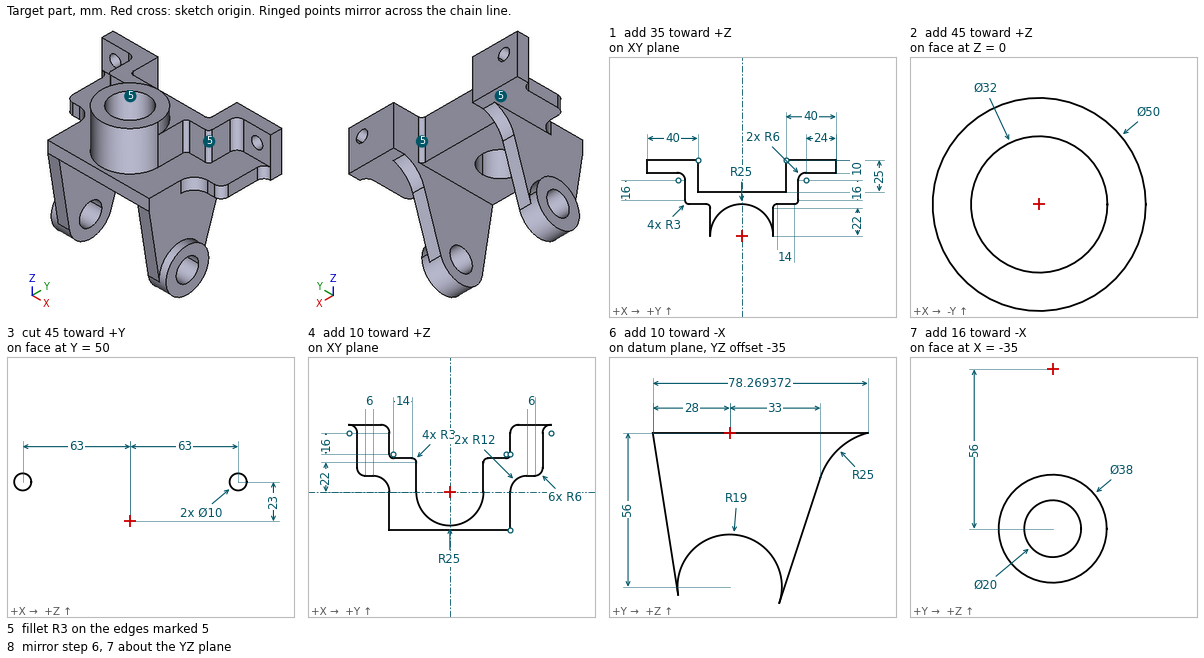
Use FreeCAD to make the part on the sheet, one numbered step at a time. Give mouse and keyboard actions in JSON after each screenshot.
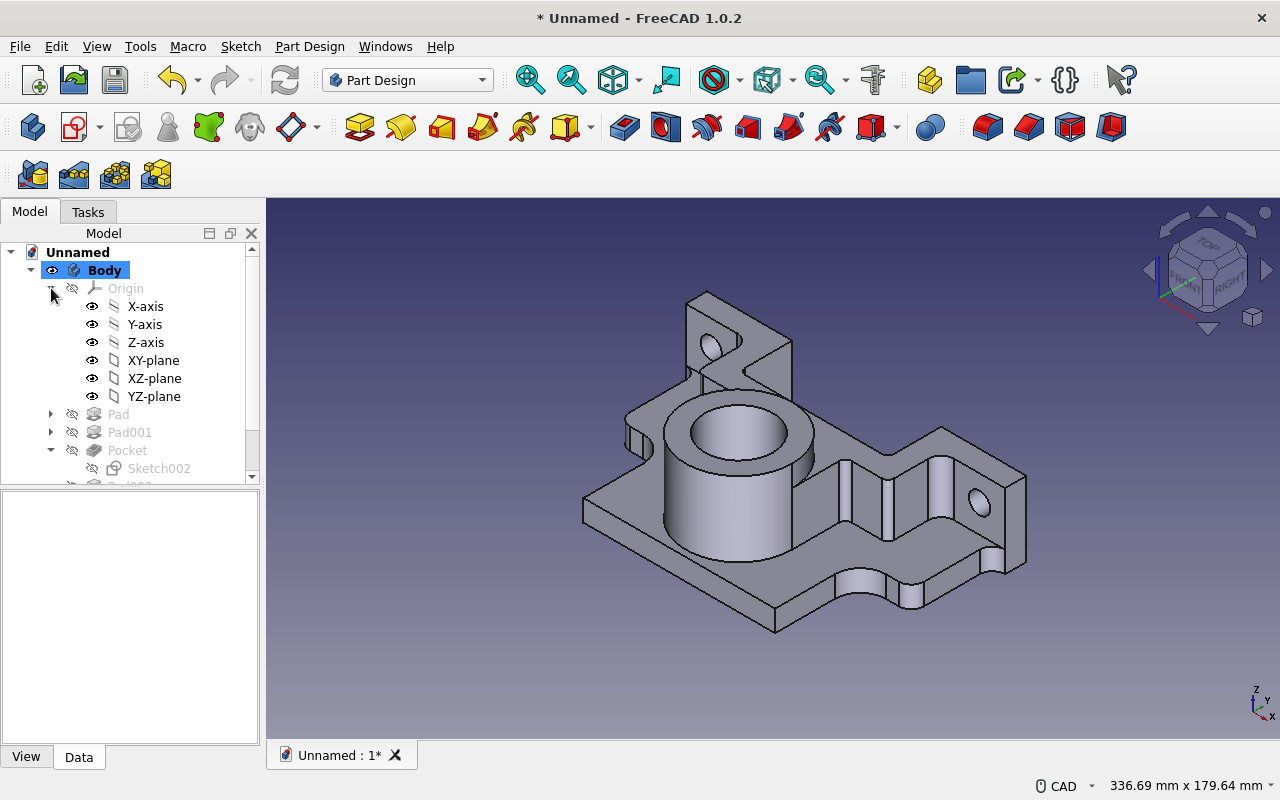
{"action": "left_click", "coordinate": [137, 396]}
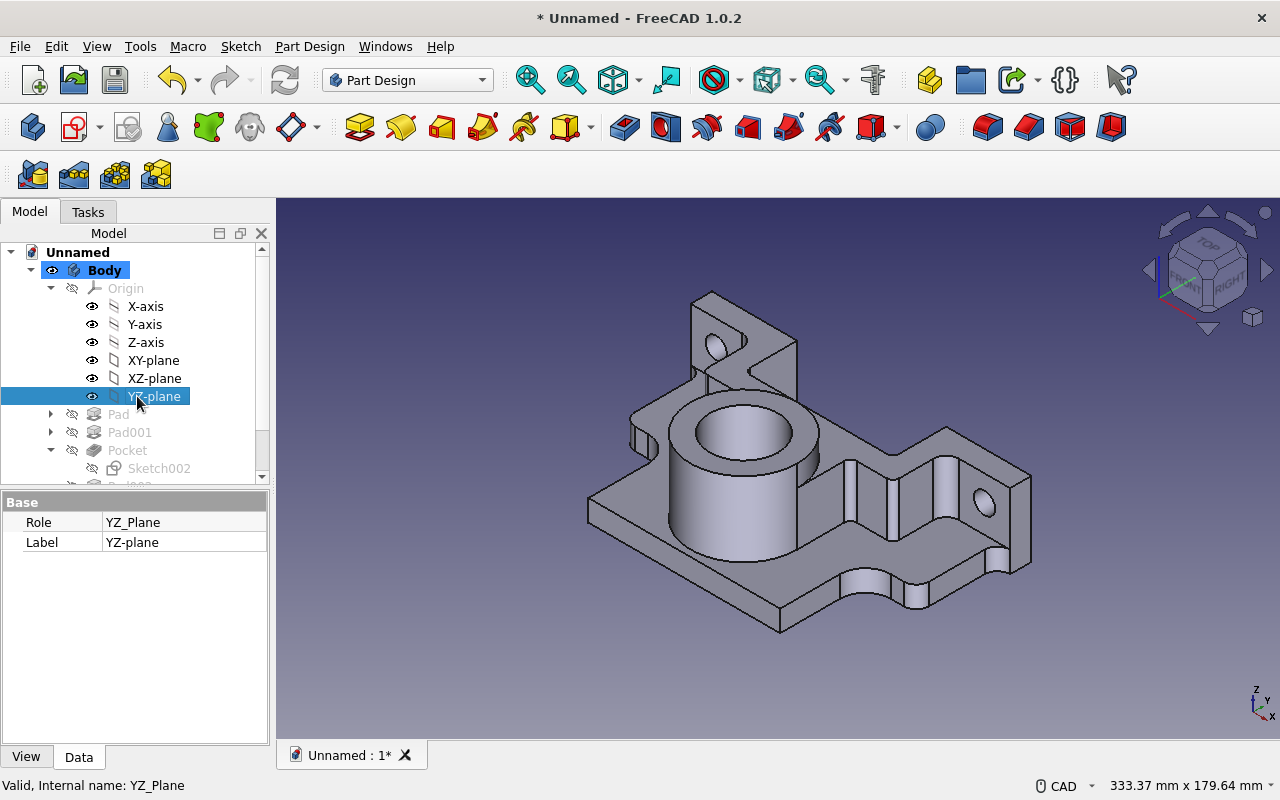
{"action": "left_click", "coordinate": [290, 128]}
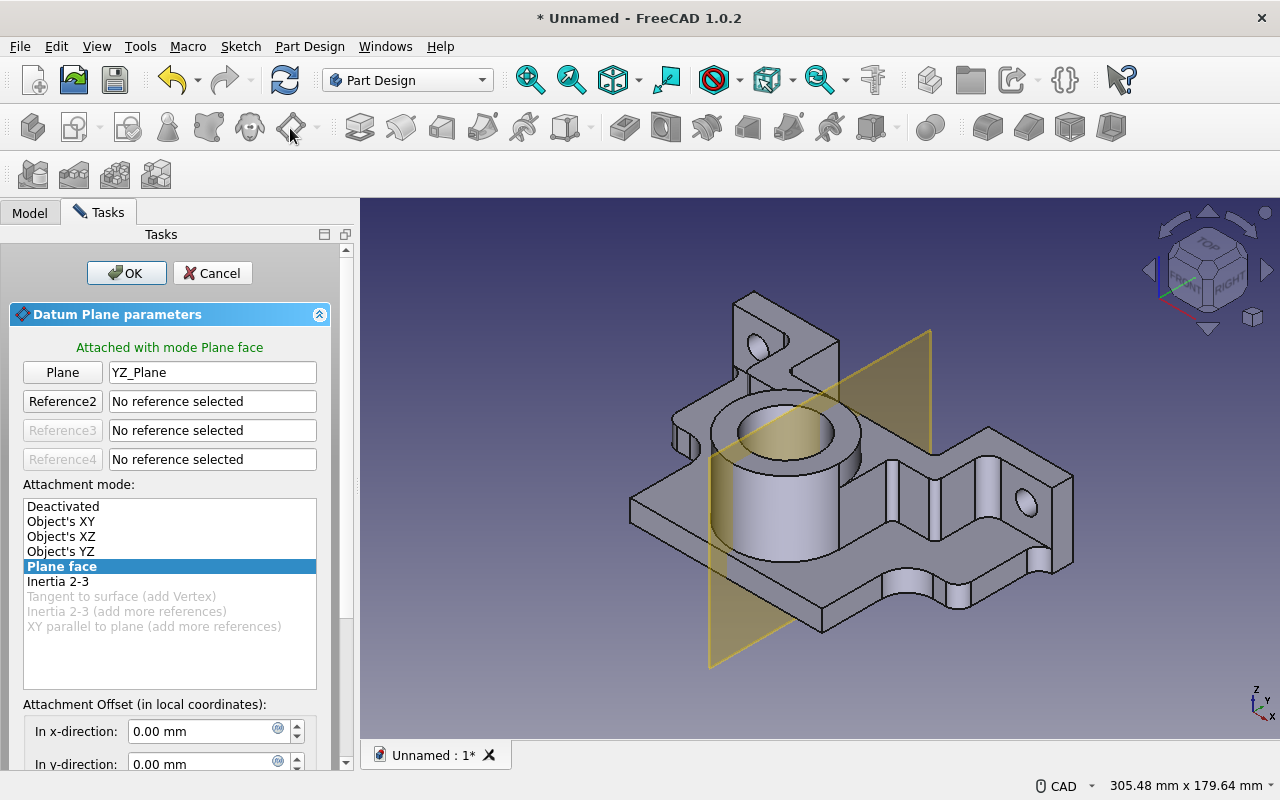
{"action": "scroll", "coordinate": [346, 507], "scroll_direction": "down", "scroll_amount": 2}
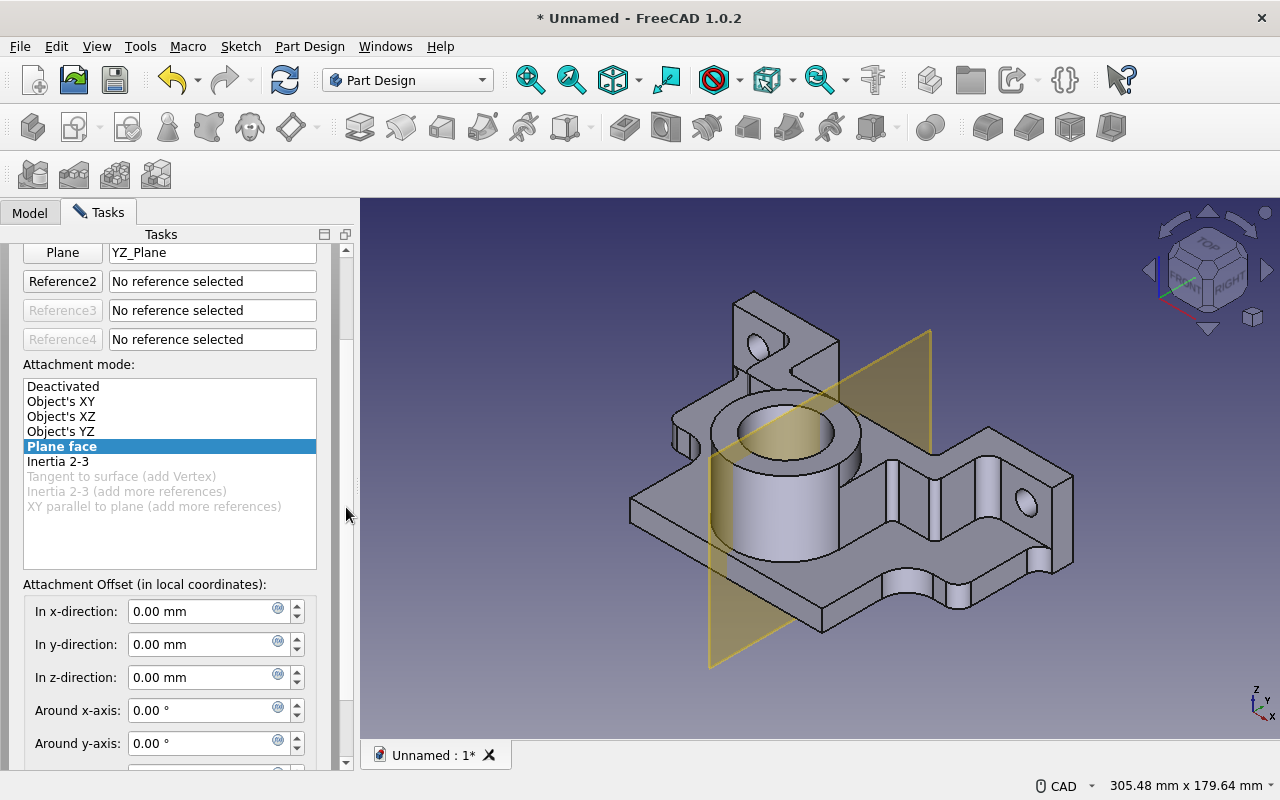
{"action": "triple_click", "coordinate": [210, 678]}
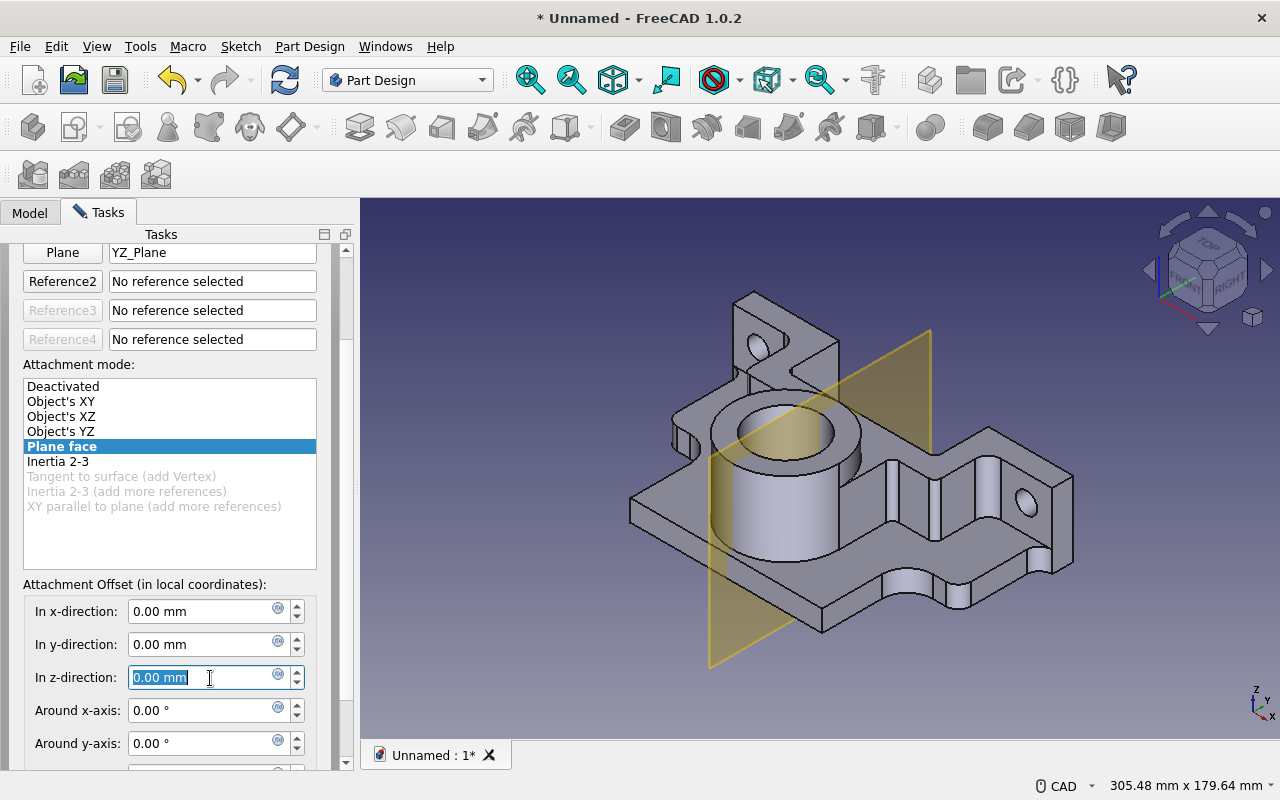
{"action": "type", "text": "-35"}
{"action": "key", "text": "Tab"}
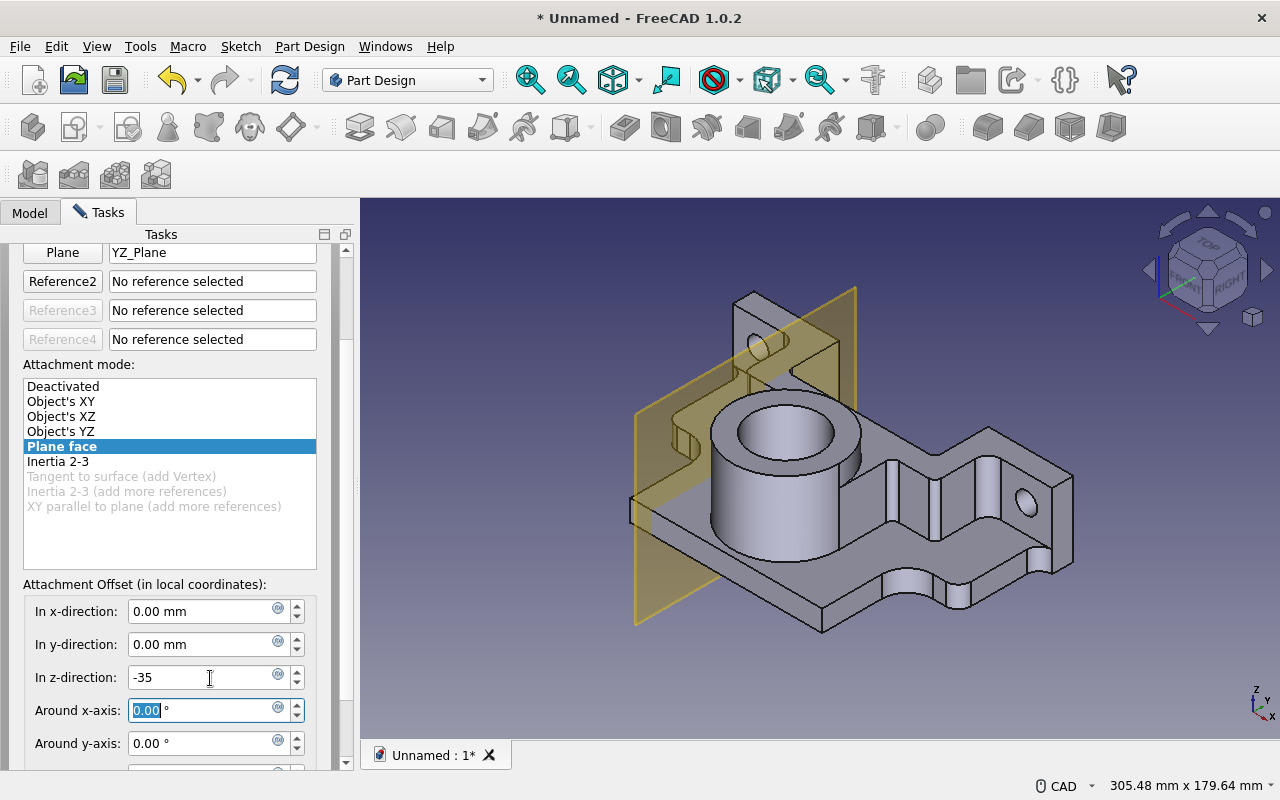
{"action": "scroll", "coordinate": [346, 507], "scroll_direction": "up", "scroll_amount": 3}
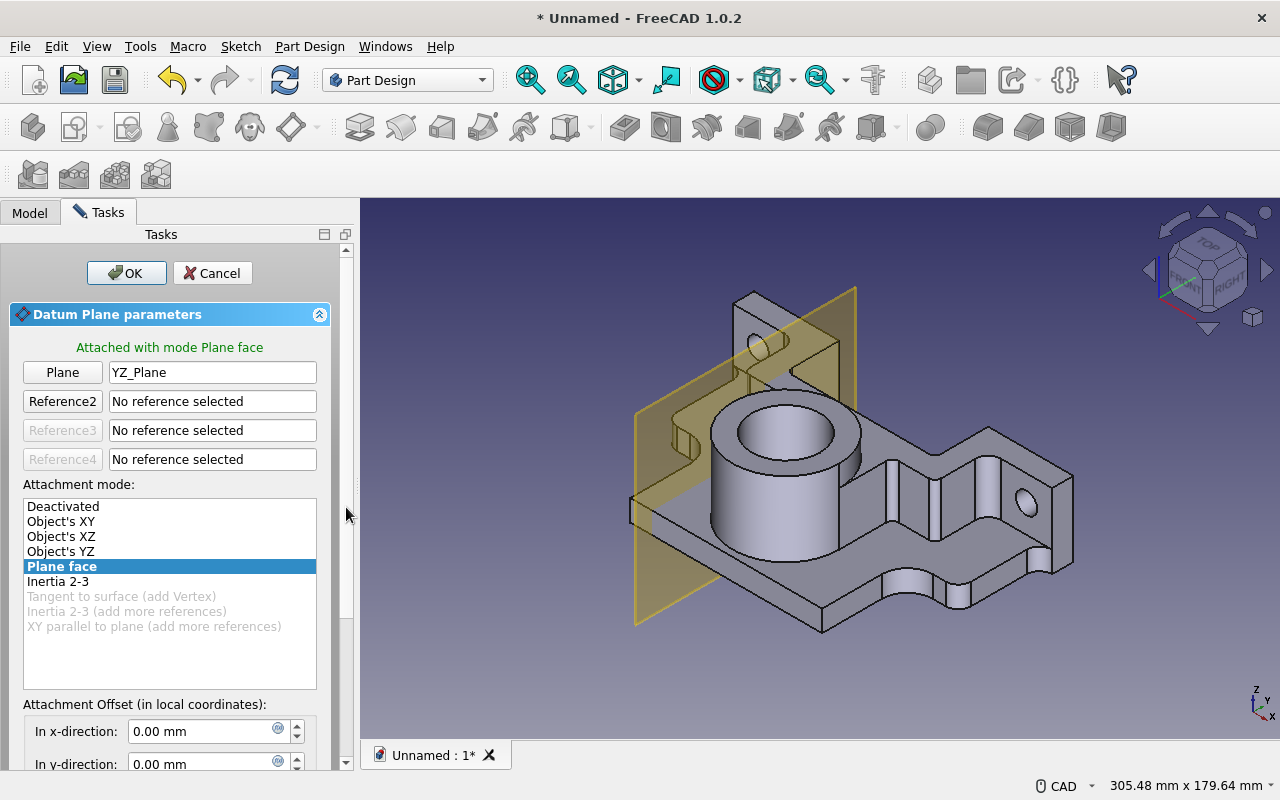
{"action": "left_click", "coordinate": [127, 273]}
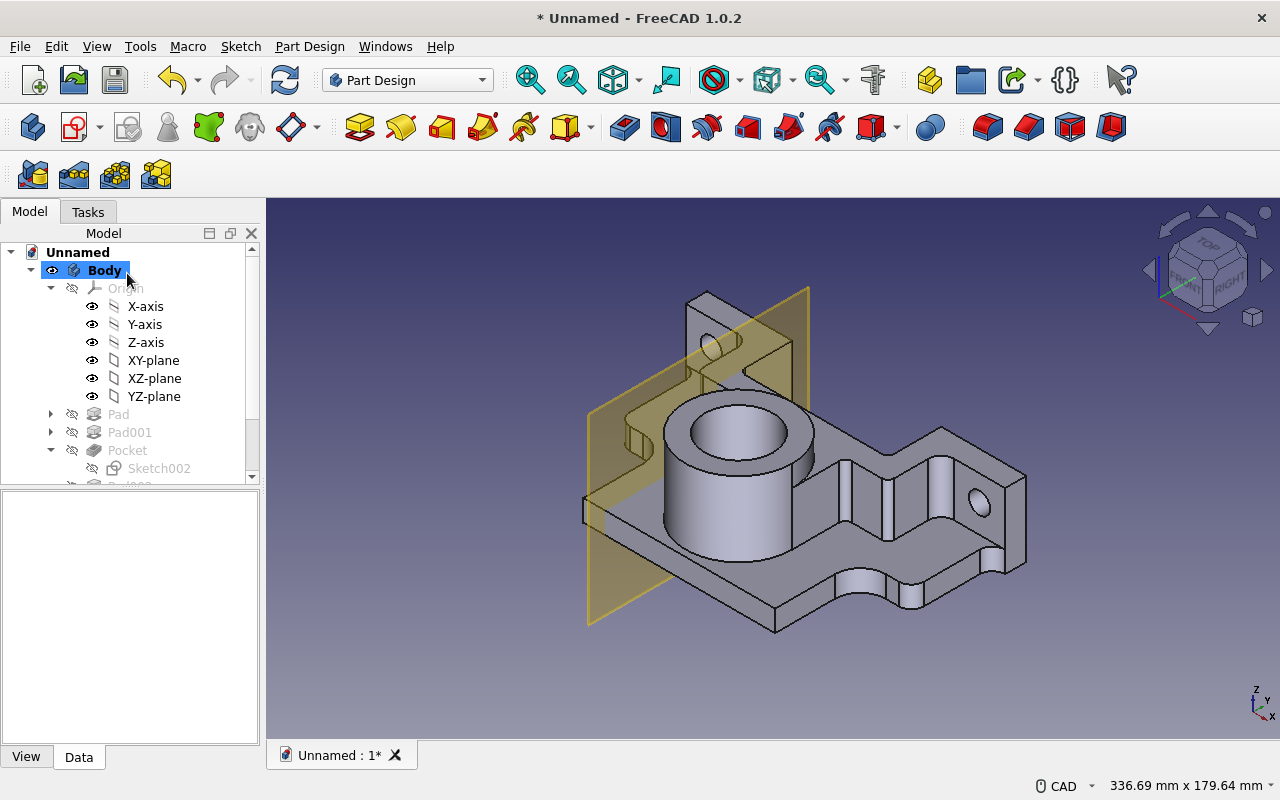
{"action": "scroll", "coordinate": [101, 356], "scroll_direction": "down", "scroll_amount": 3}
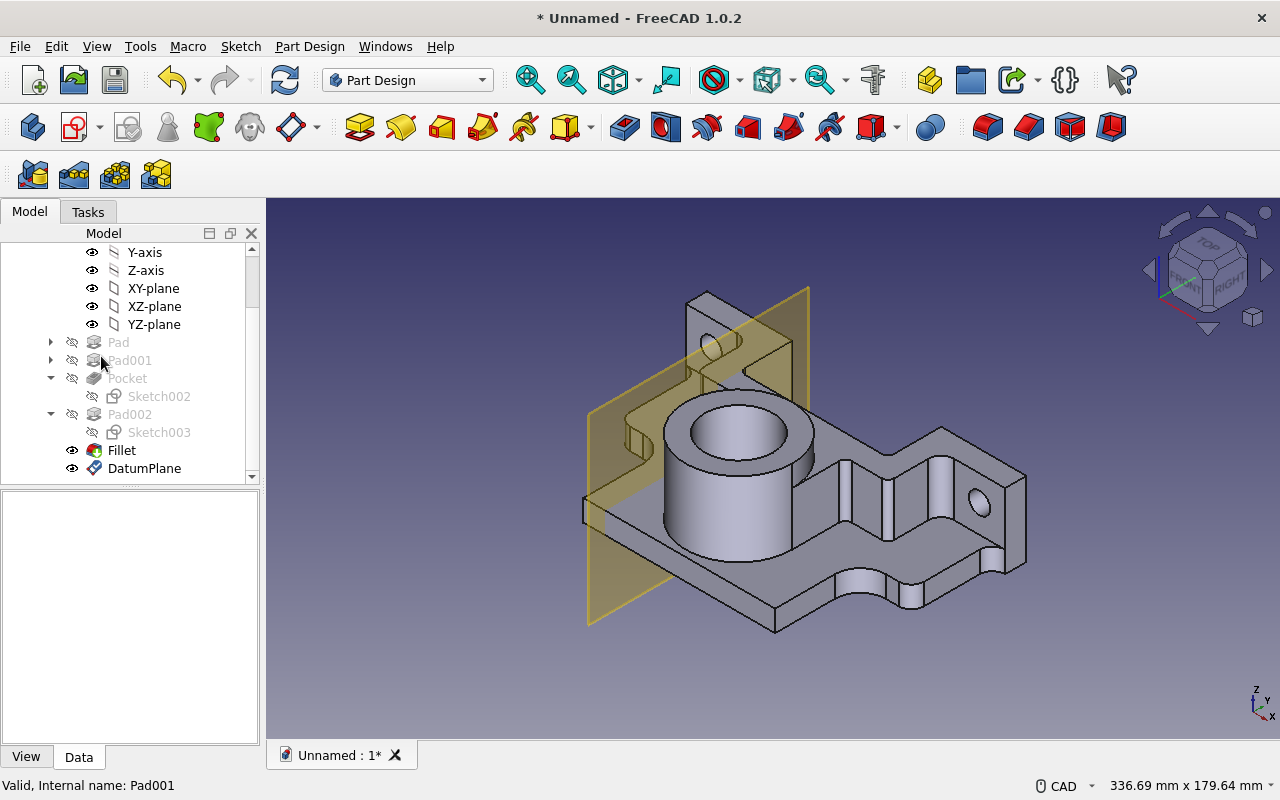
{"action": "left_click", "coordinate": [117, 468]}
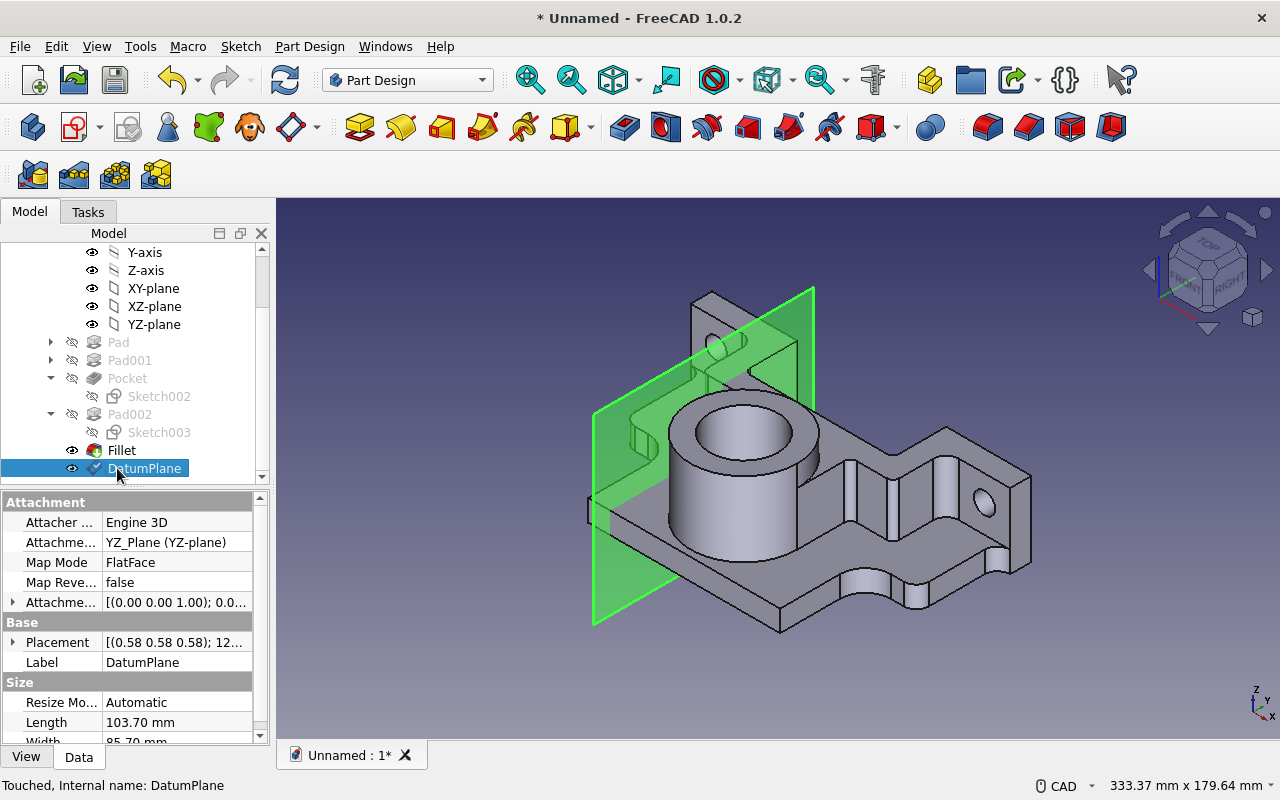
{"action": "left_click", "coordinate": [74, 128]}